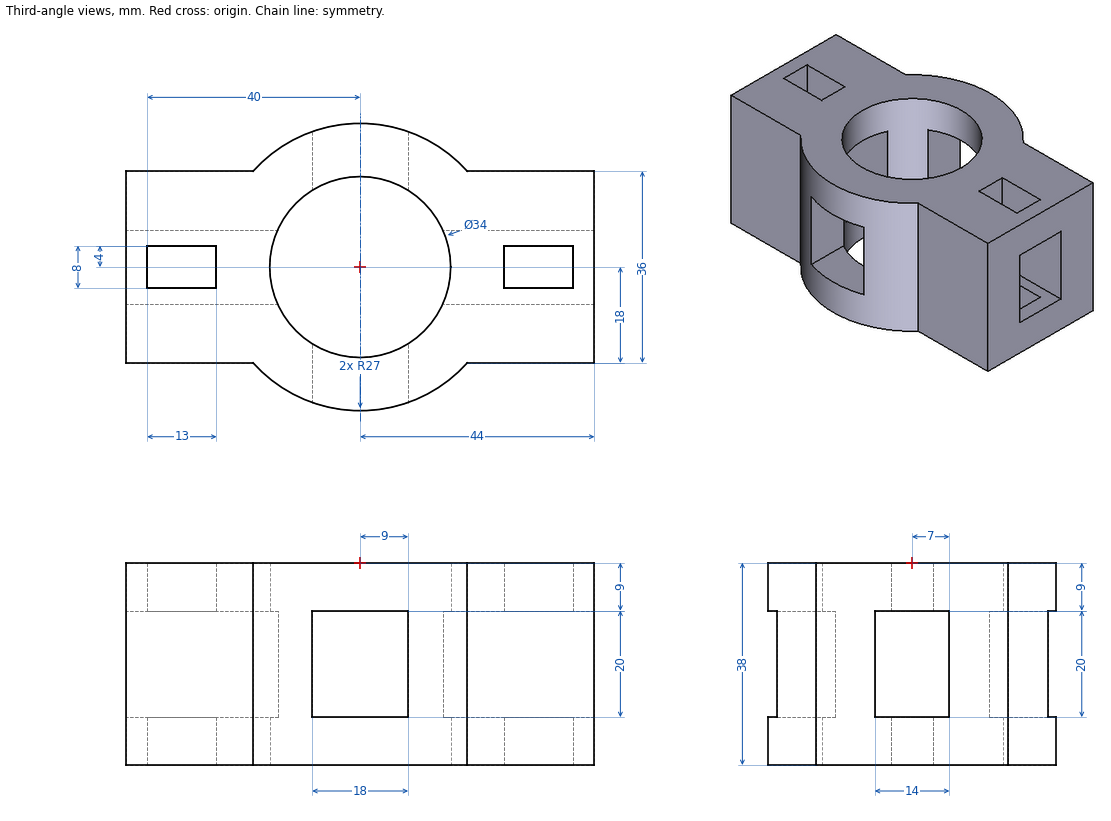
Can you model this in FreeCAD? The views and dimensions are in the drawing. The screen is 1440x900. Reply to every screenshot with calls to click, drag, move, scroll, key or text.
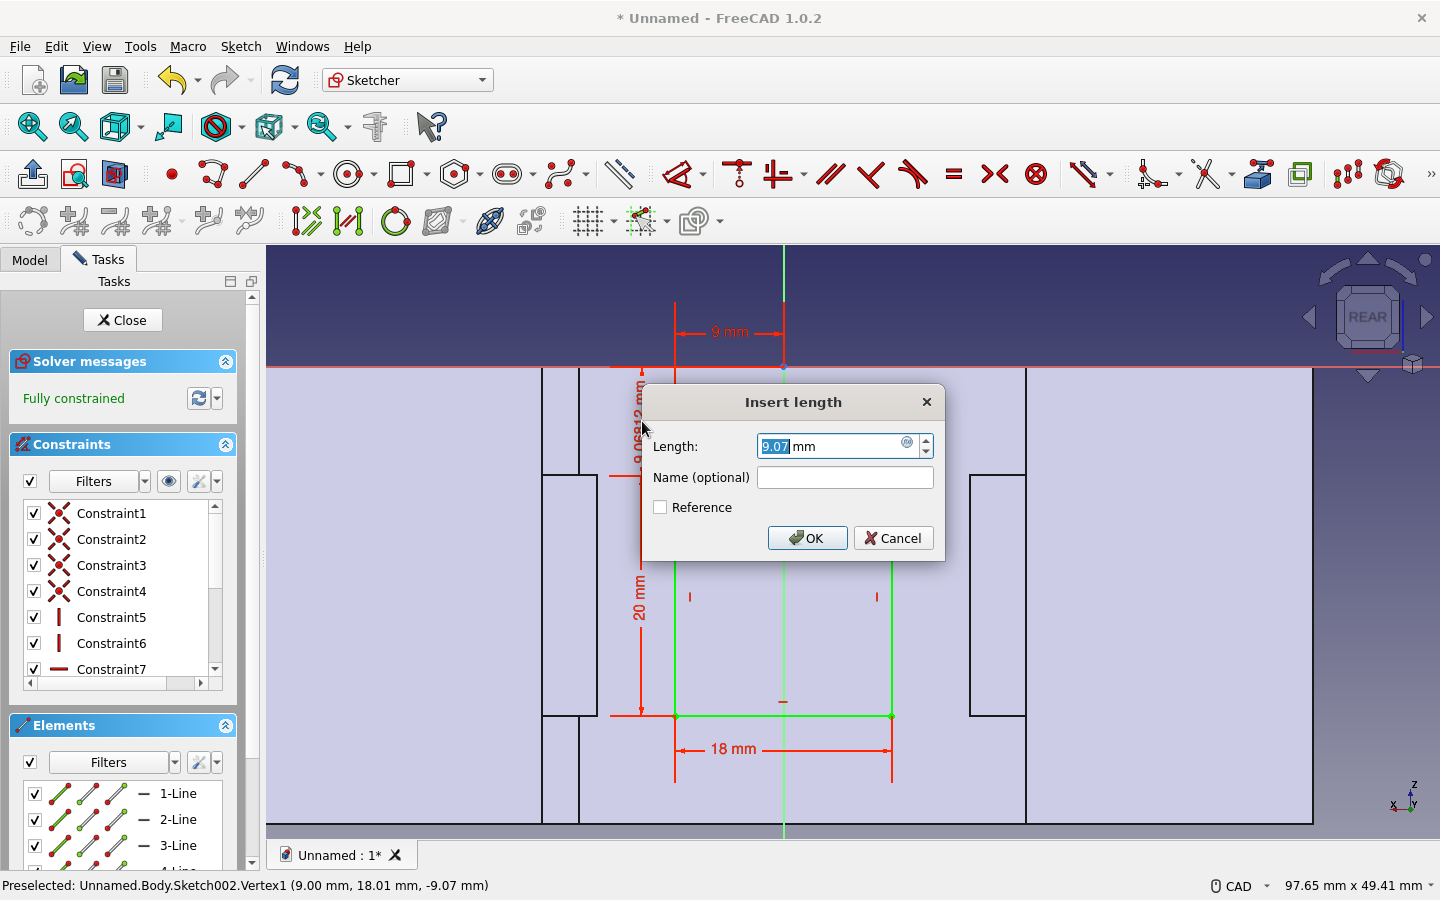
text(9)
key(Return)
key(Escape)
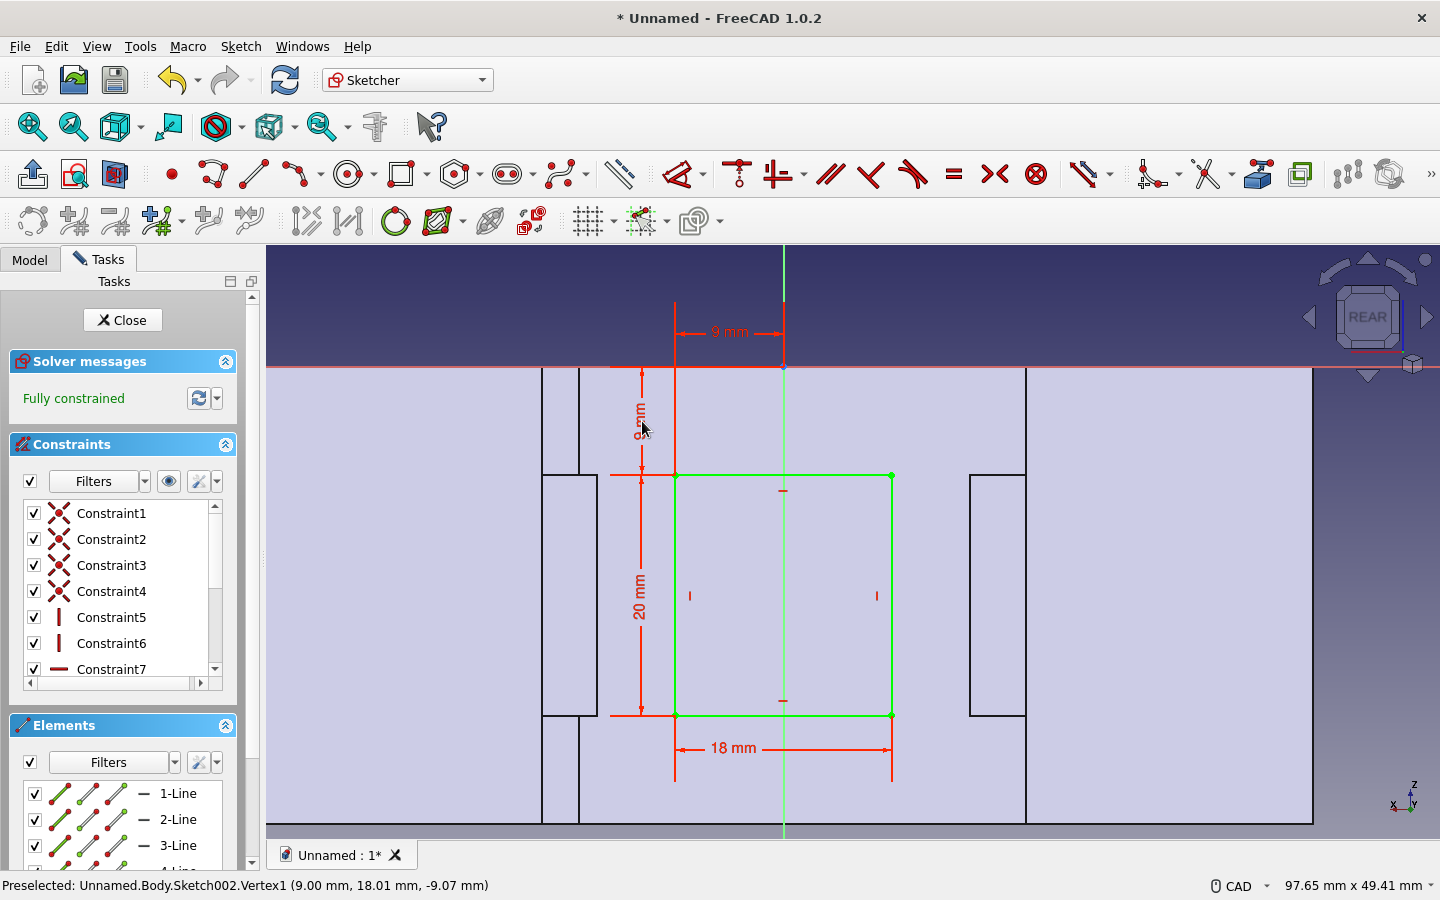
click(123, 320)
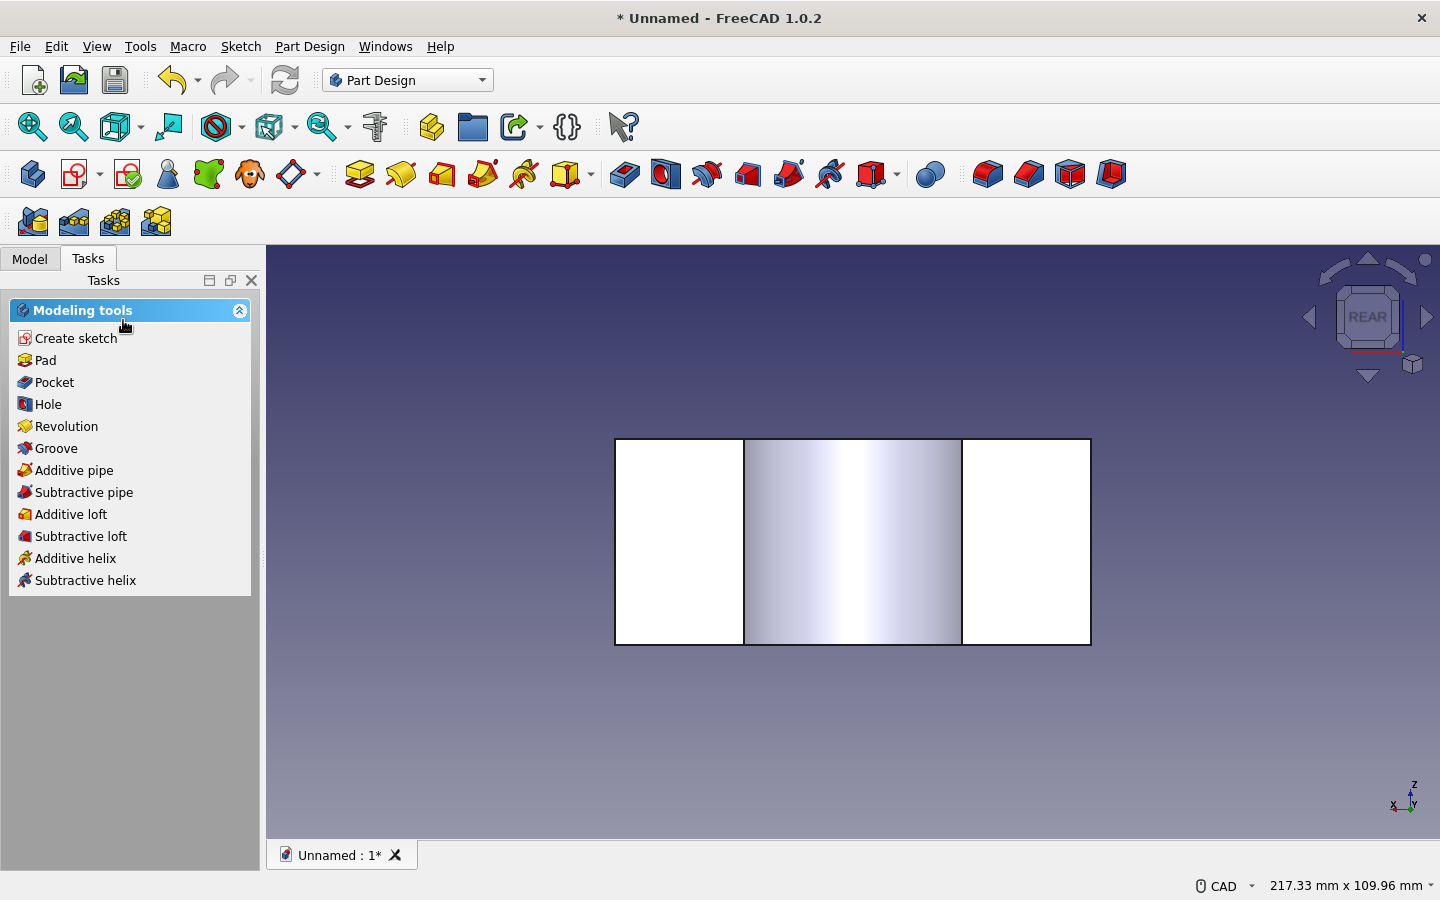
click(625, 174)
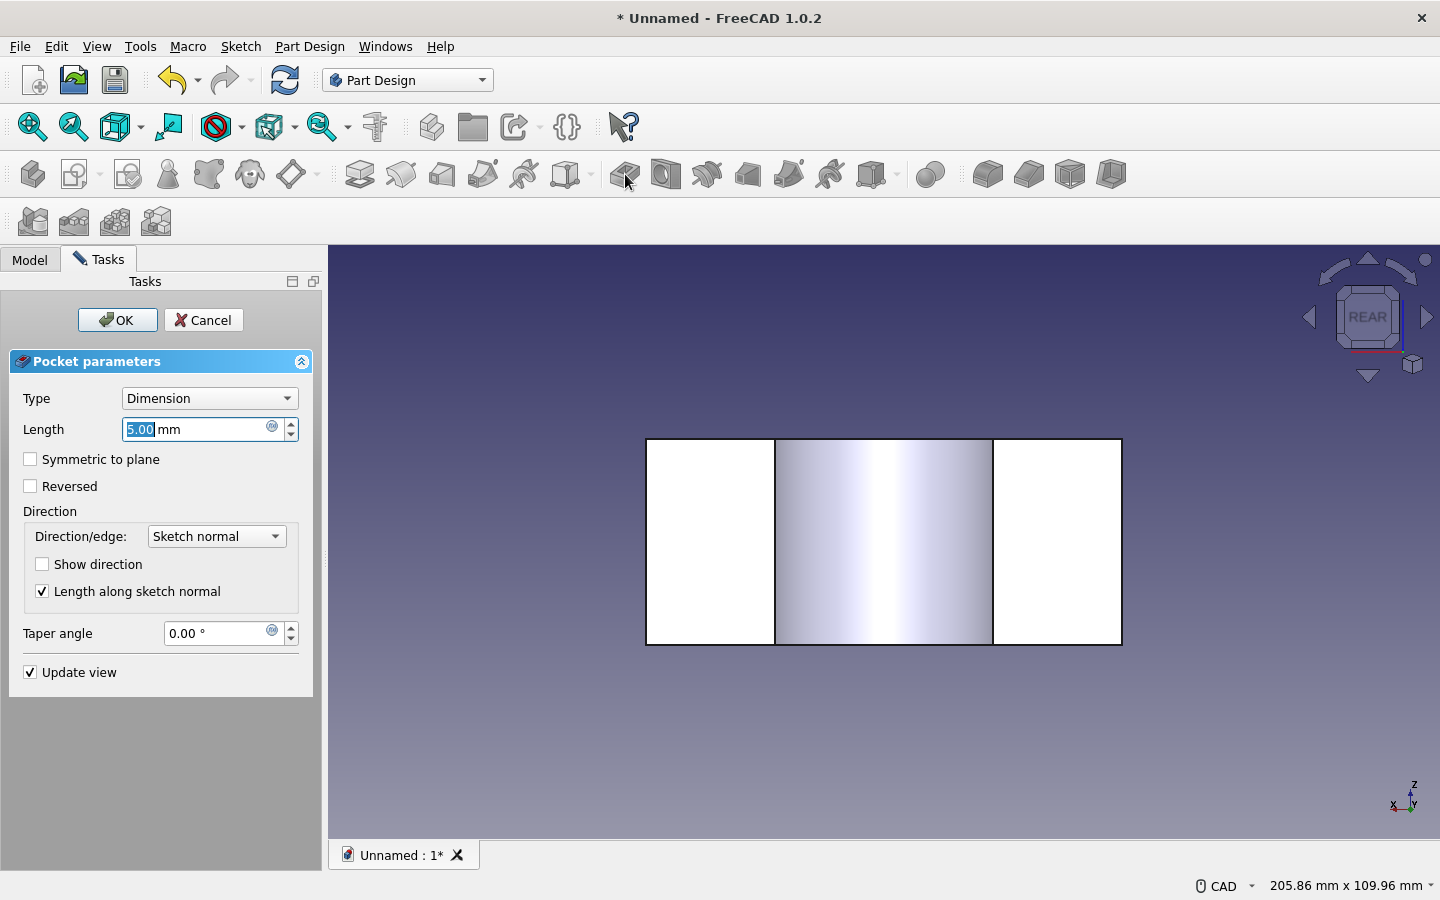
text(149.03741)
key(Tab)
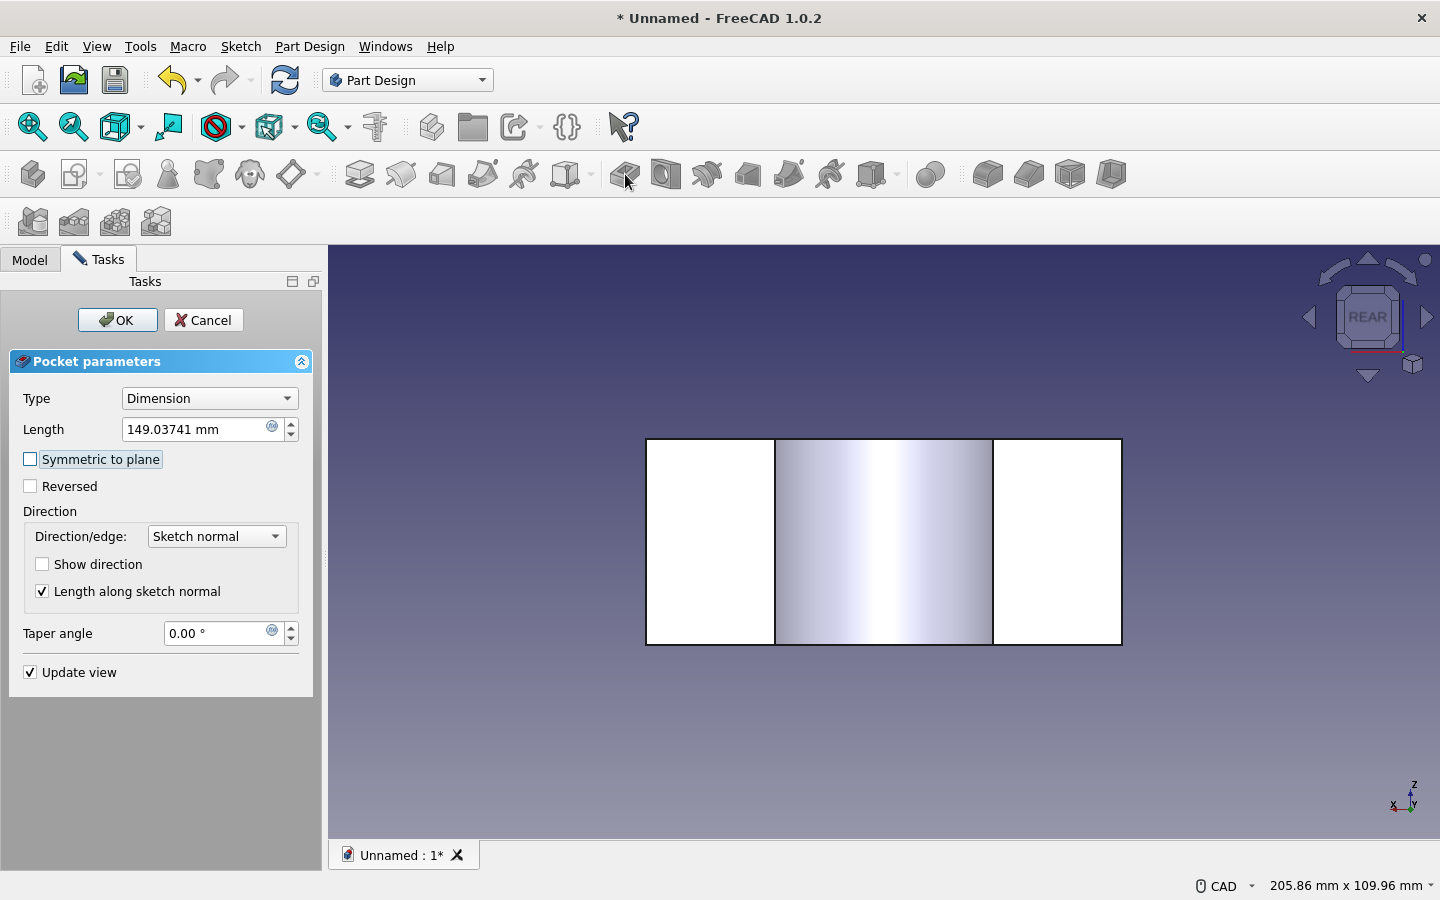
click(31, 459)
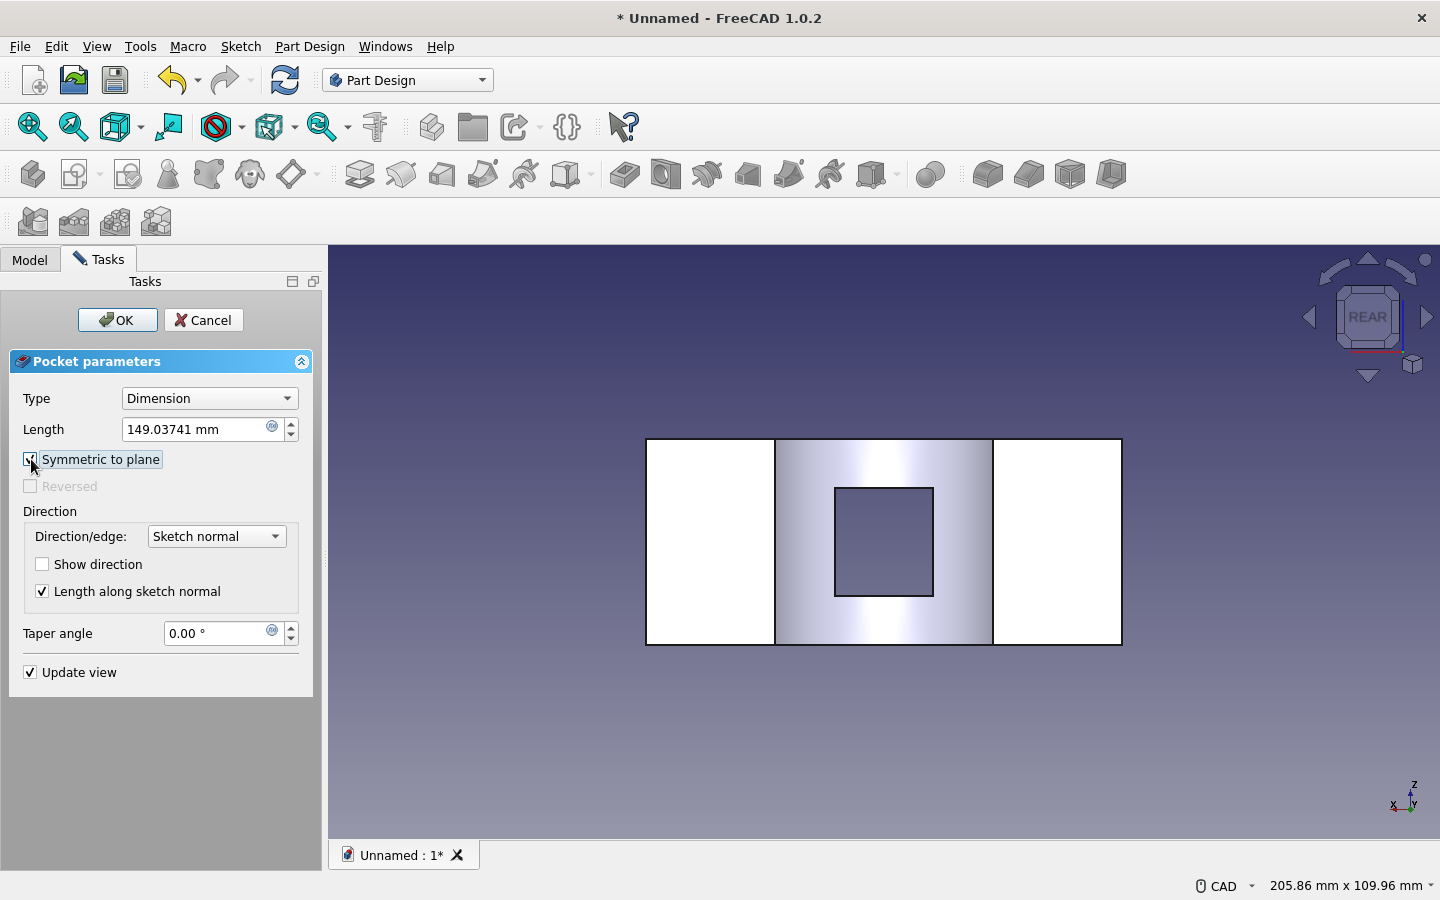
click(118, 320)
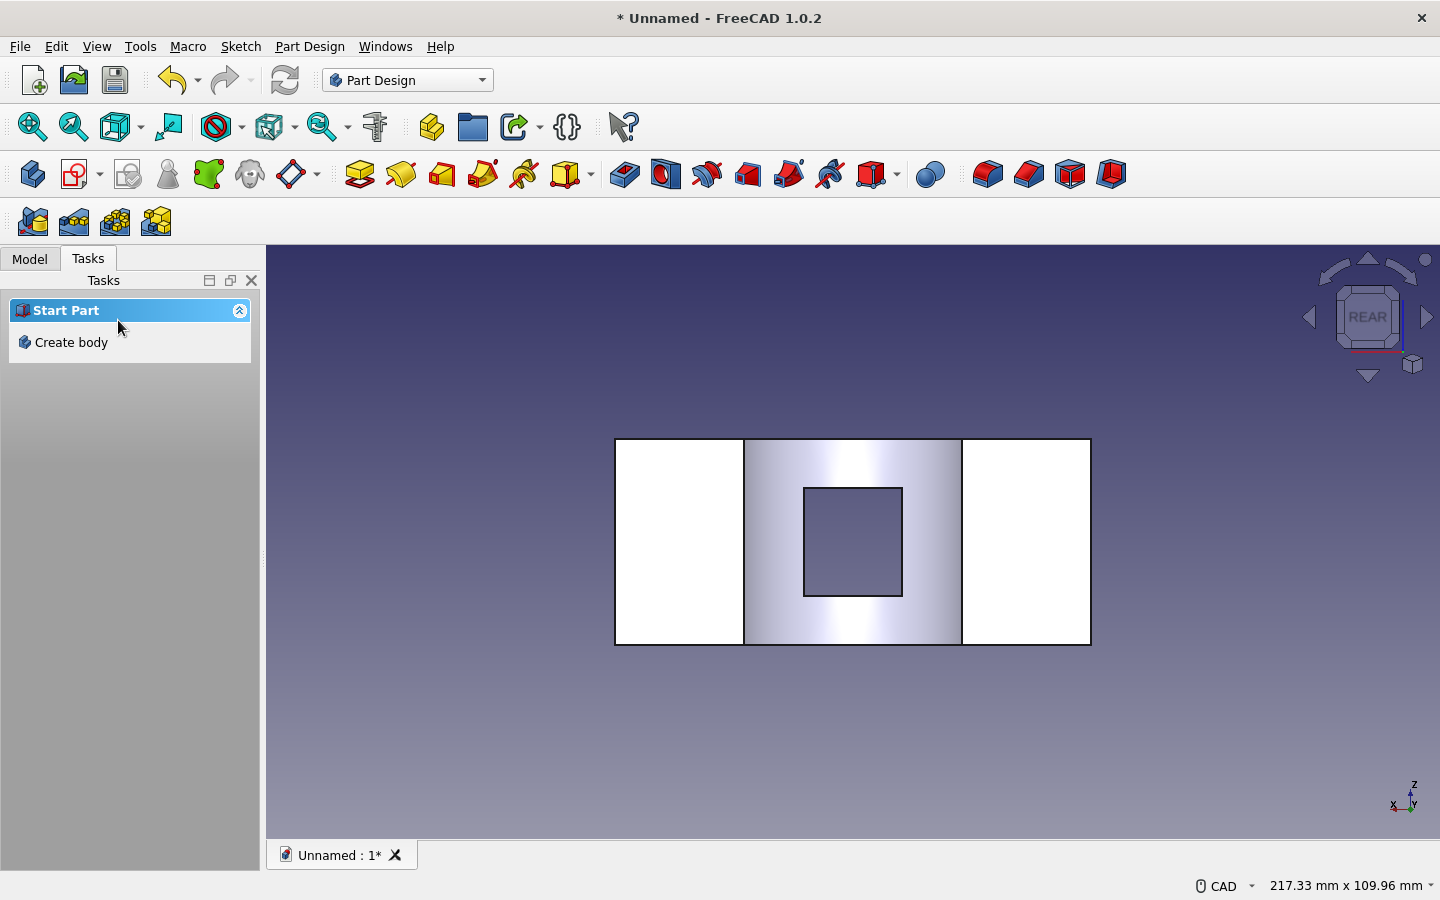
key(0)